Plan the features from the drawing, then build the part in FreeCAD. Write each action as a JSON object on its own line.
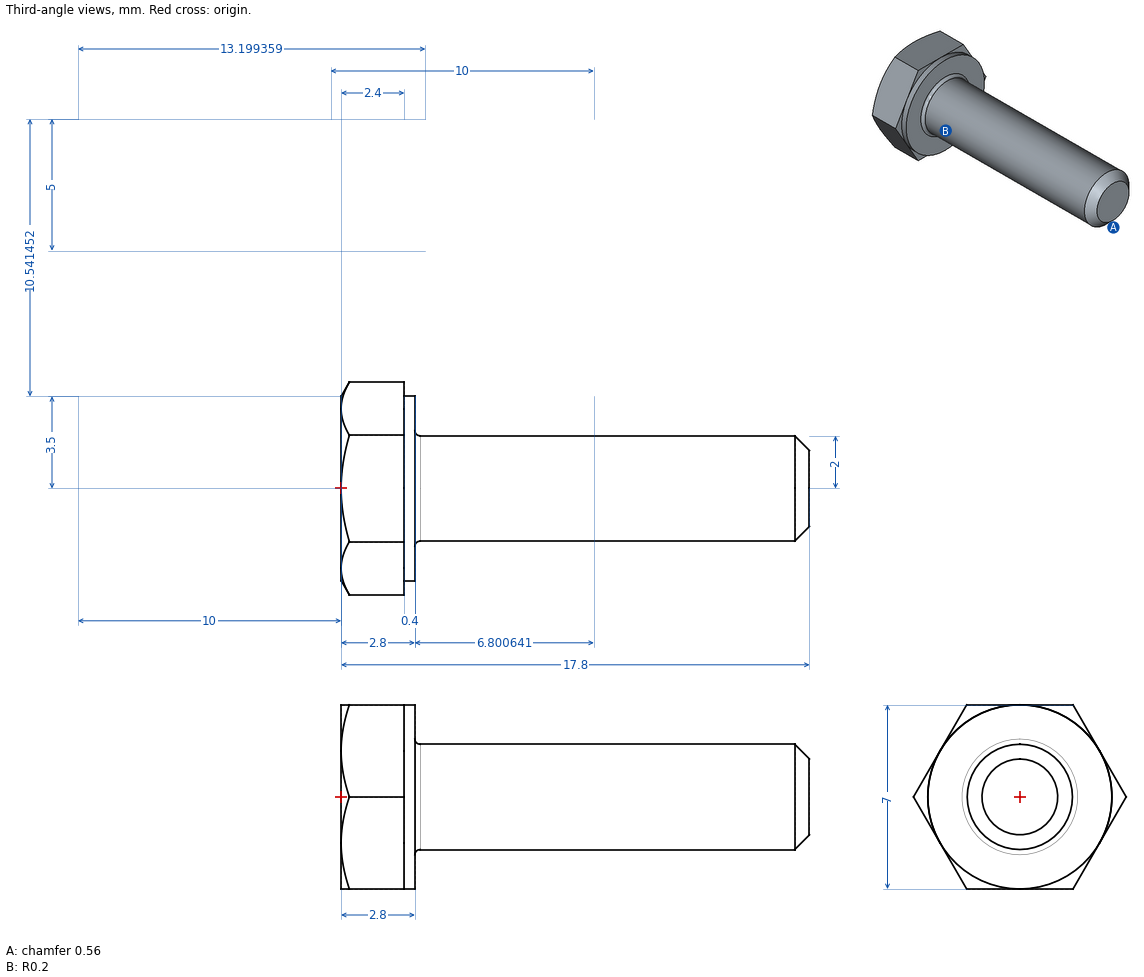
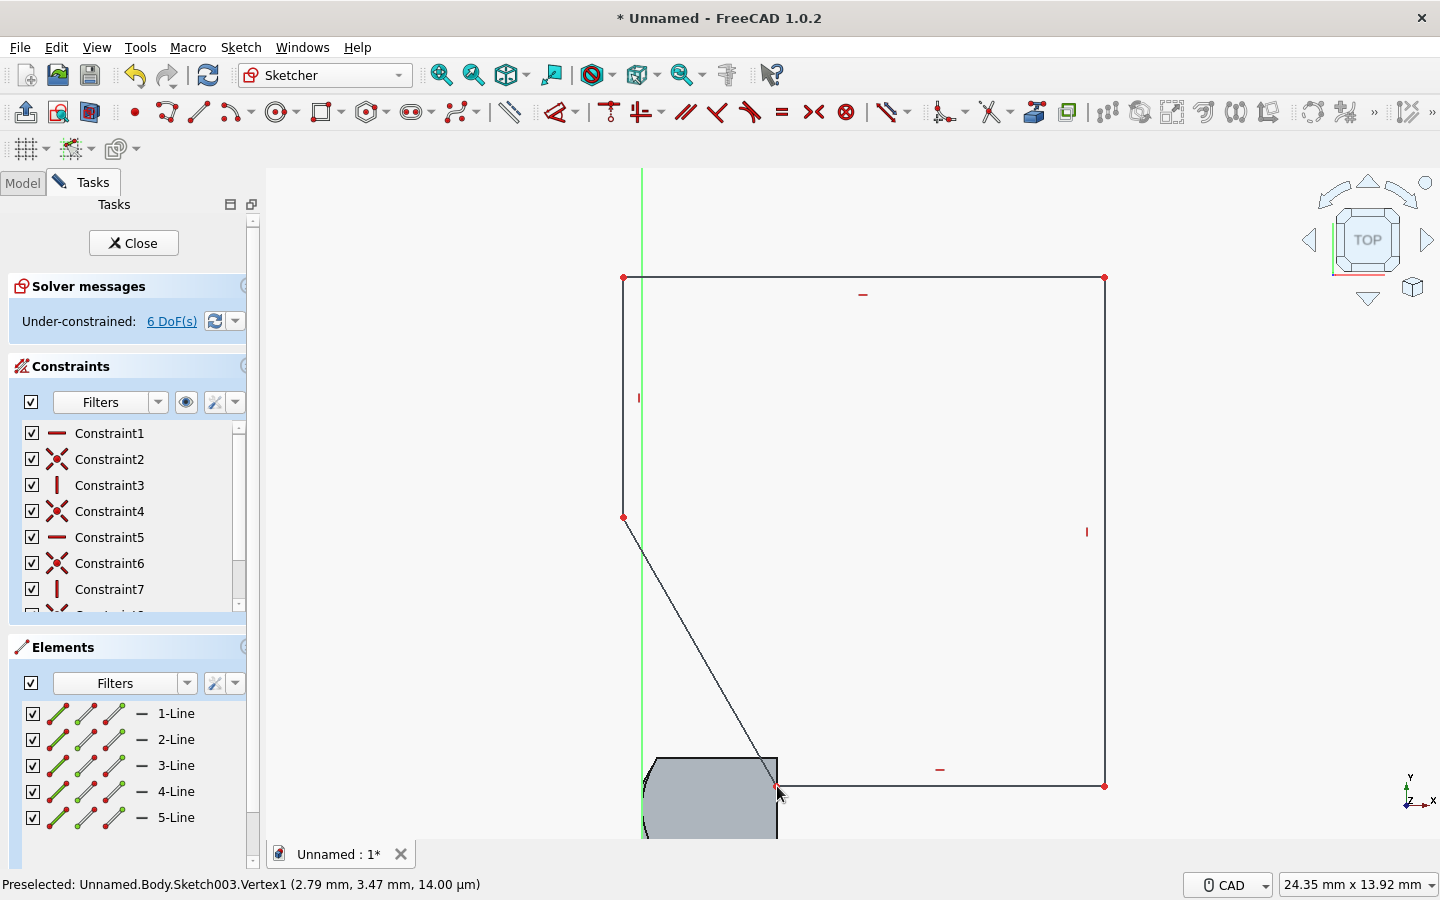
{"action": "key", "text": "d"}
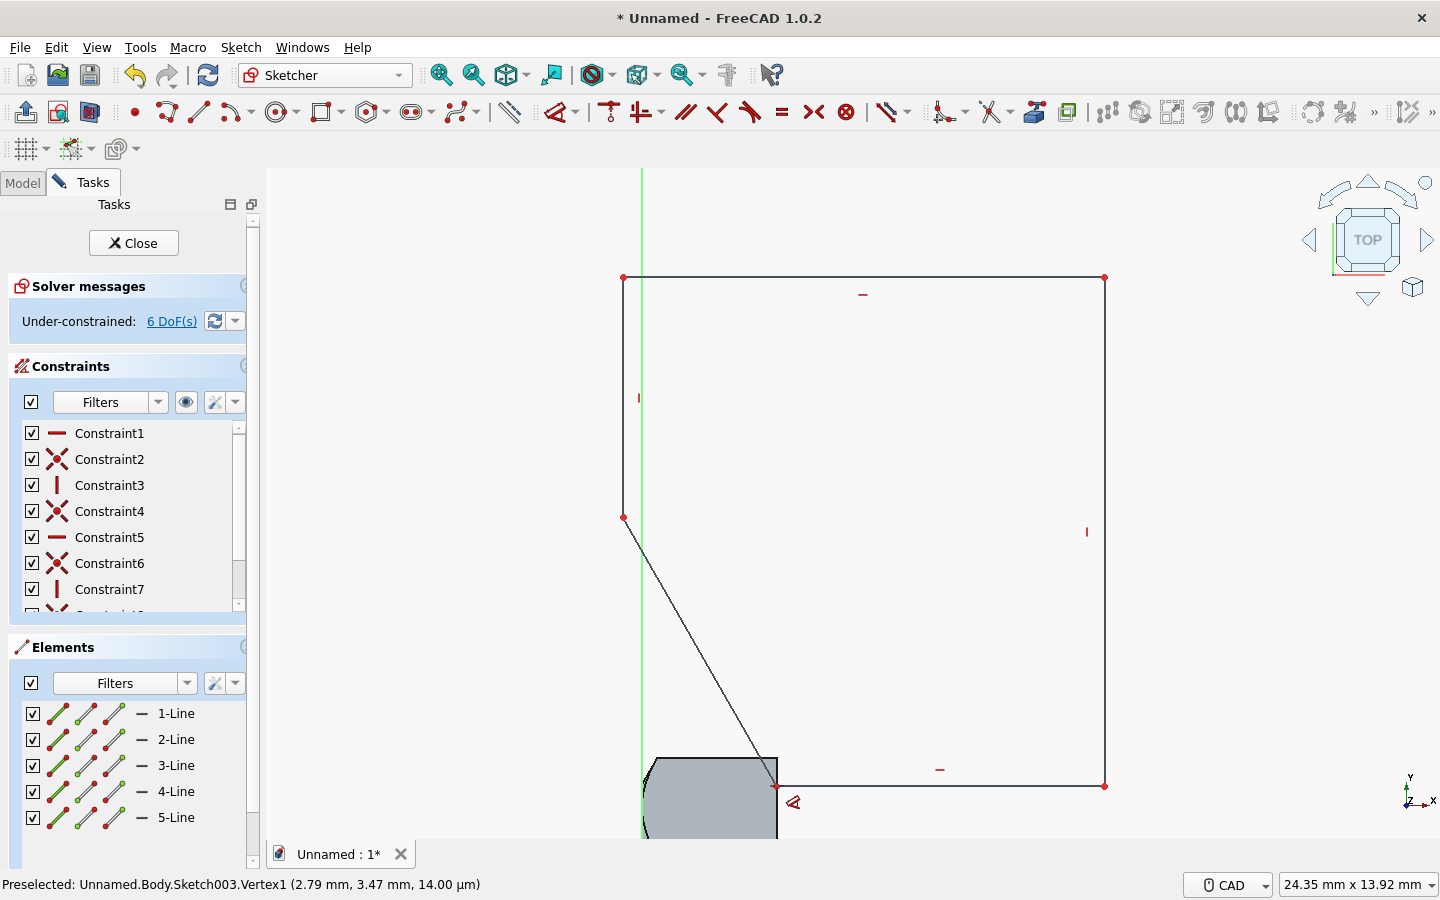
{"action": "left_click", "coordinate": [623, 350]}
{"action": "left_click", "coordinate": [589, 398]}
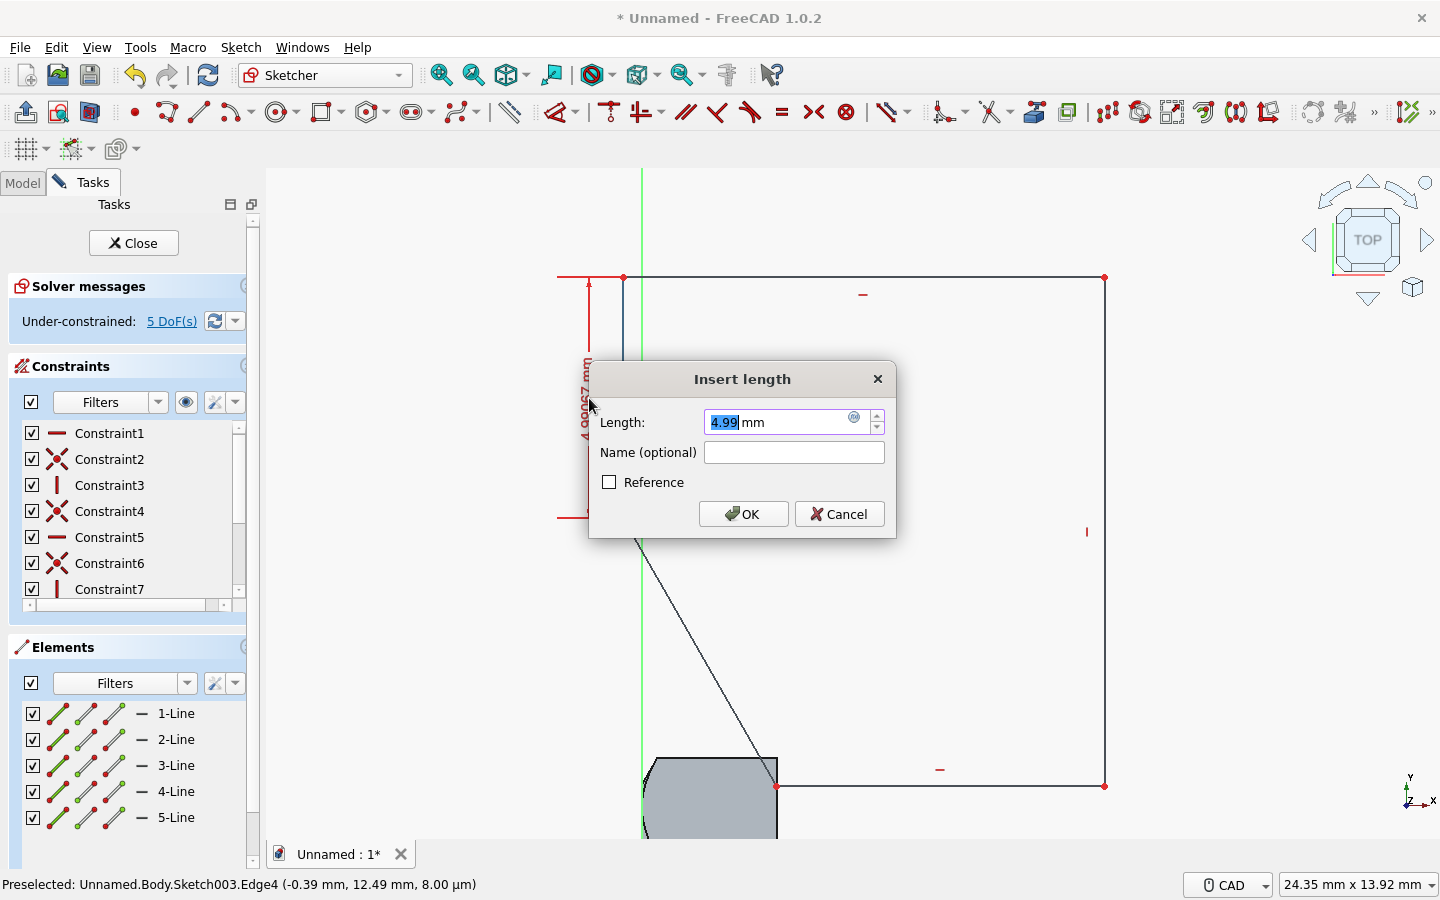
{"action": "type", "text": "5"}
{"action": "key", "text": "Return"}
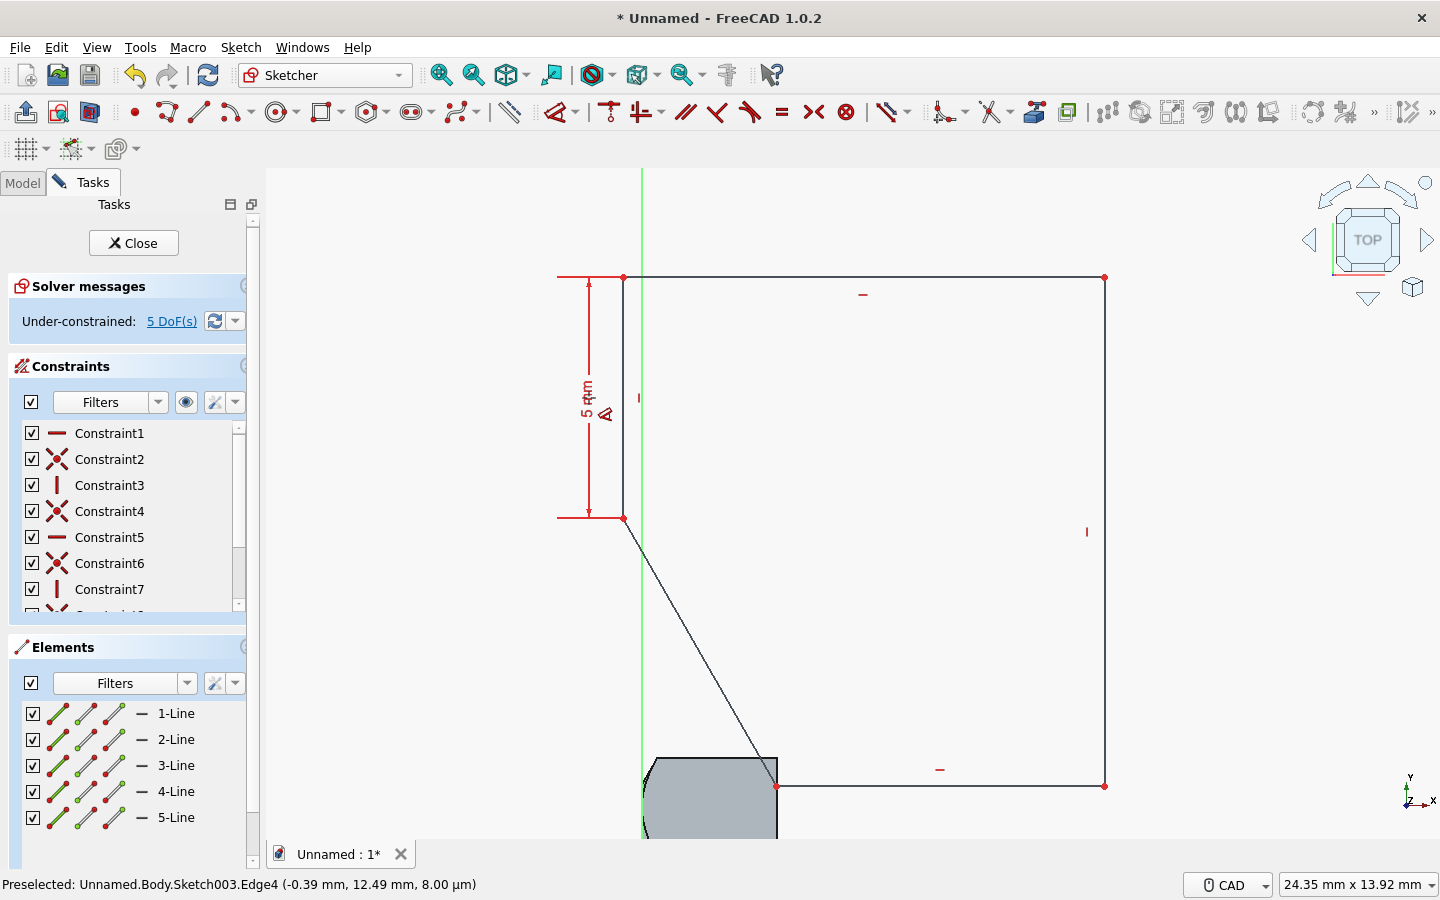
{"action": "left_click", "coordinate": [960, 277]}
{"action": "left_click", "coordinate": [864, 243]}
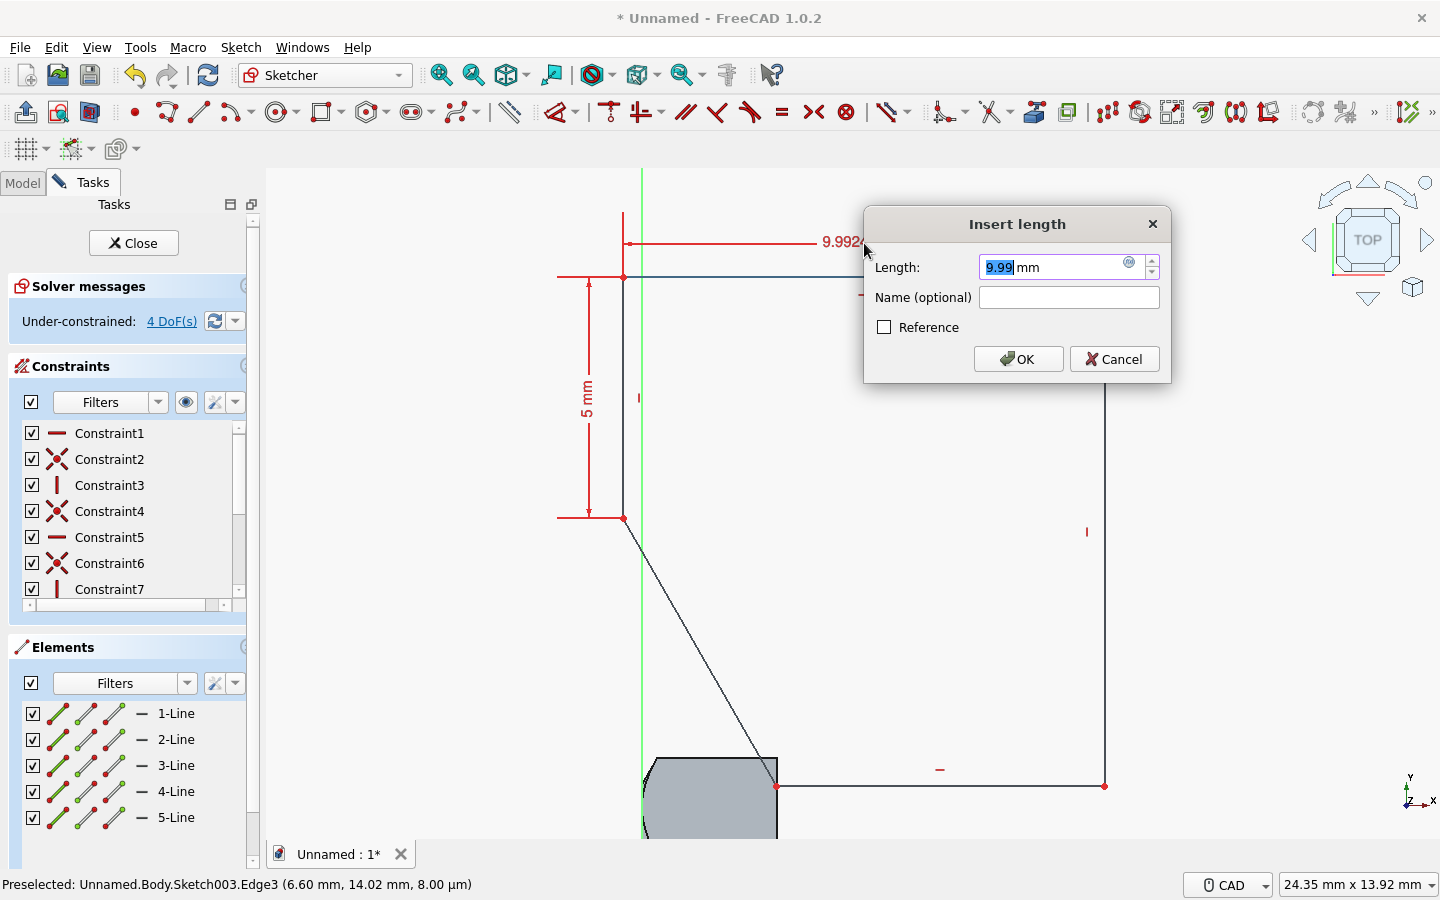
{"action": "type", "text": "10"}
{"action": "key", "text": "Return"}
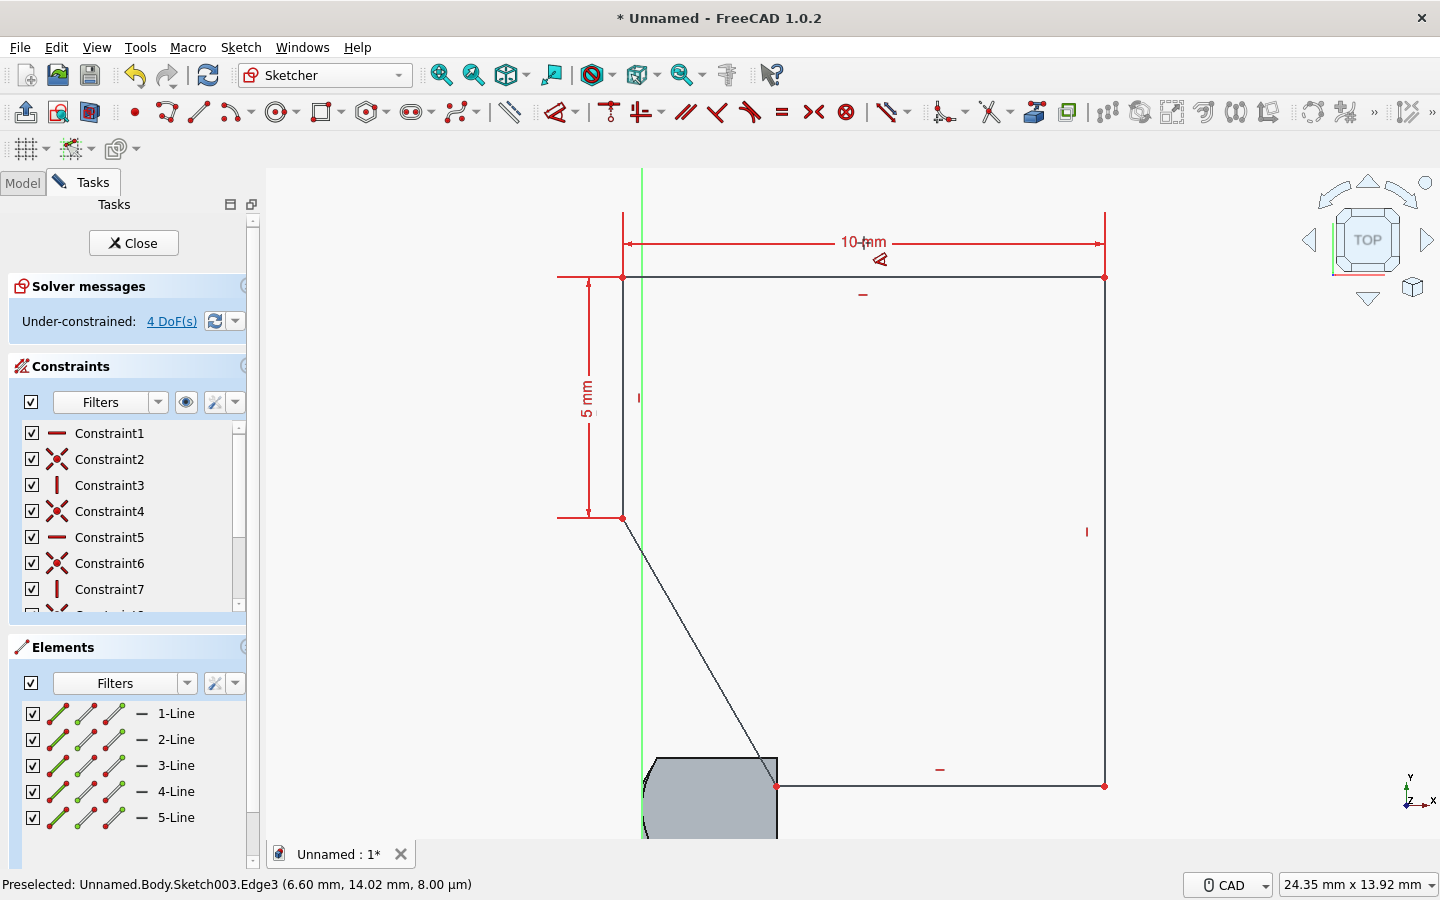
{"action": "left_click", "coordinate": [777, 786]}
{"action": "left_click", "coordinate": [709, 752]}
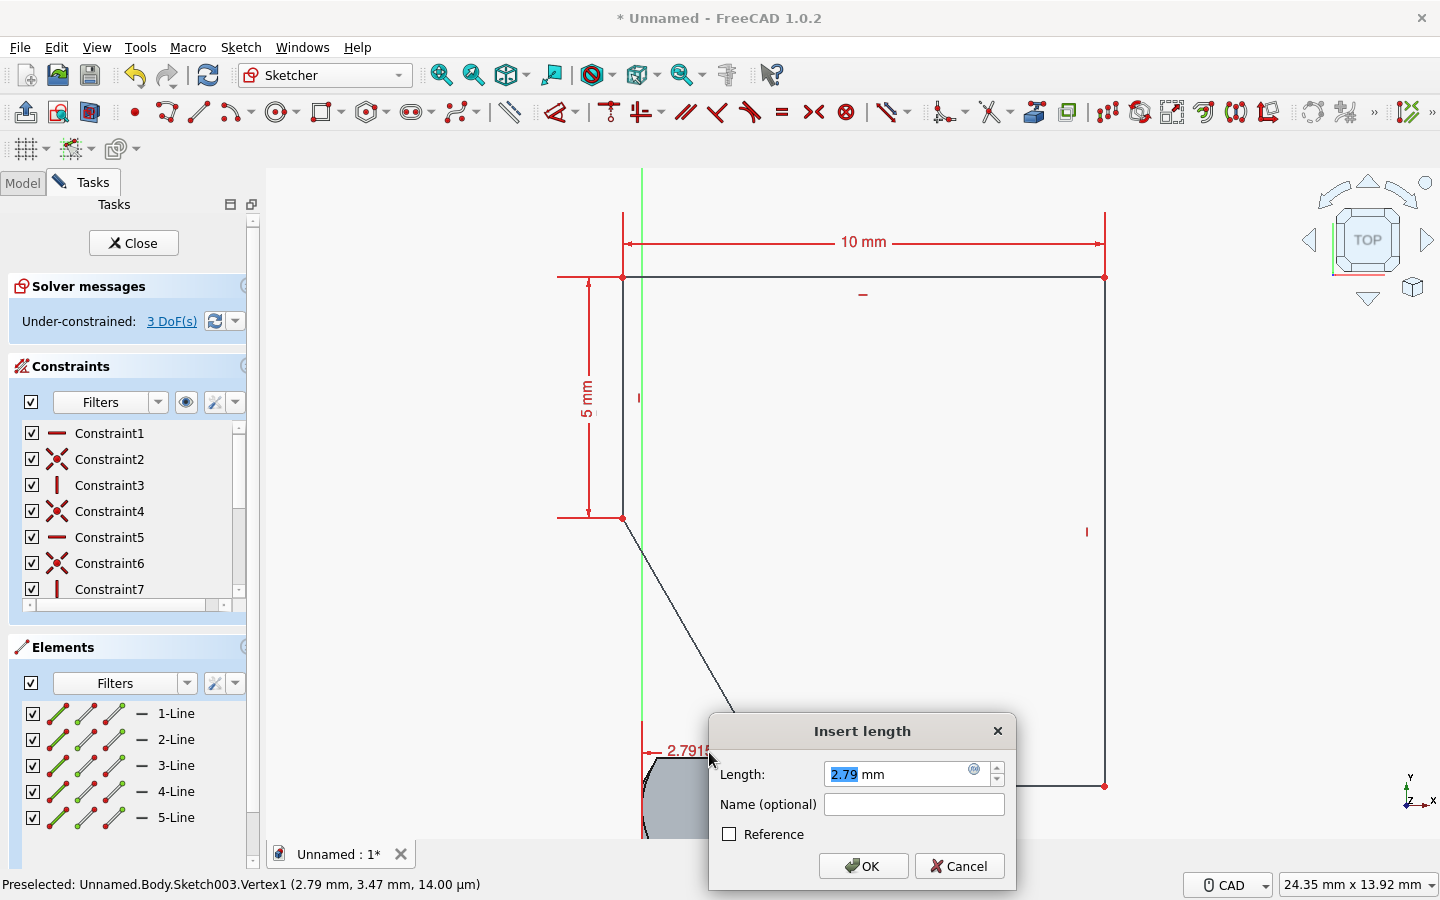
{"action": "type", "text": "2.8"}
{"action": "key", "text": "Return"}